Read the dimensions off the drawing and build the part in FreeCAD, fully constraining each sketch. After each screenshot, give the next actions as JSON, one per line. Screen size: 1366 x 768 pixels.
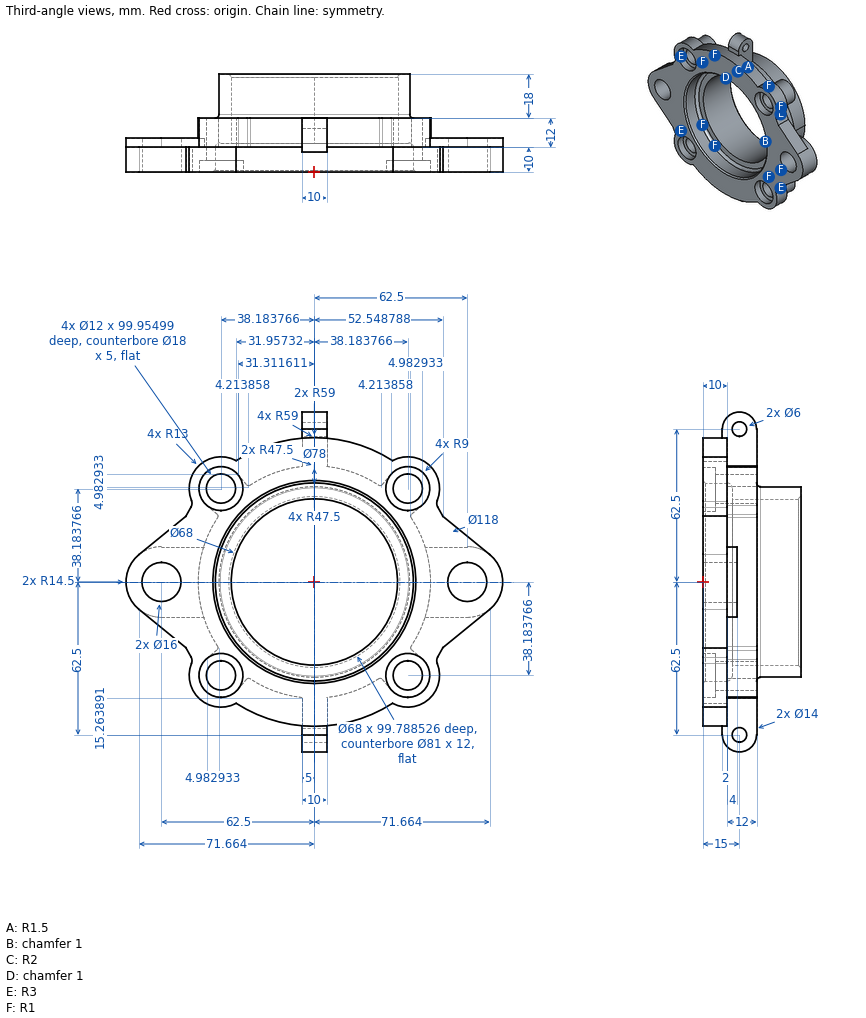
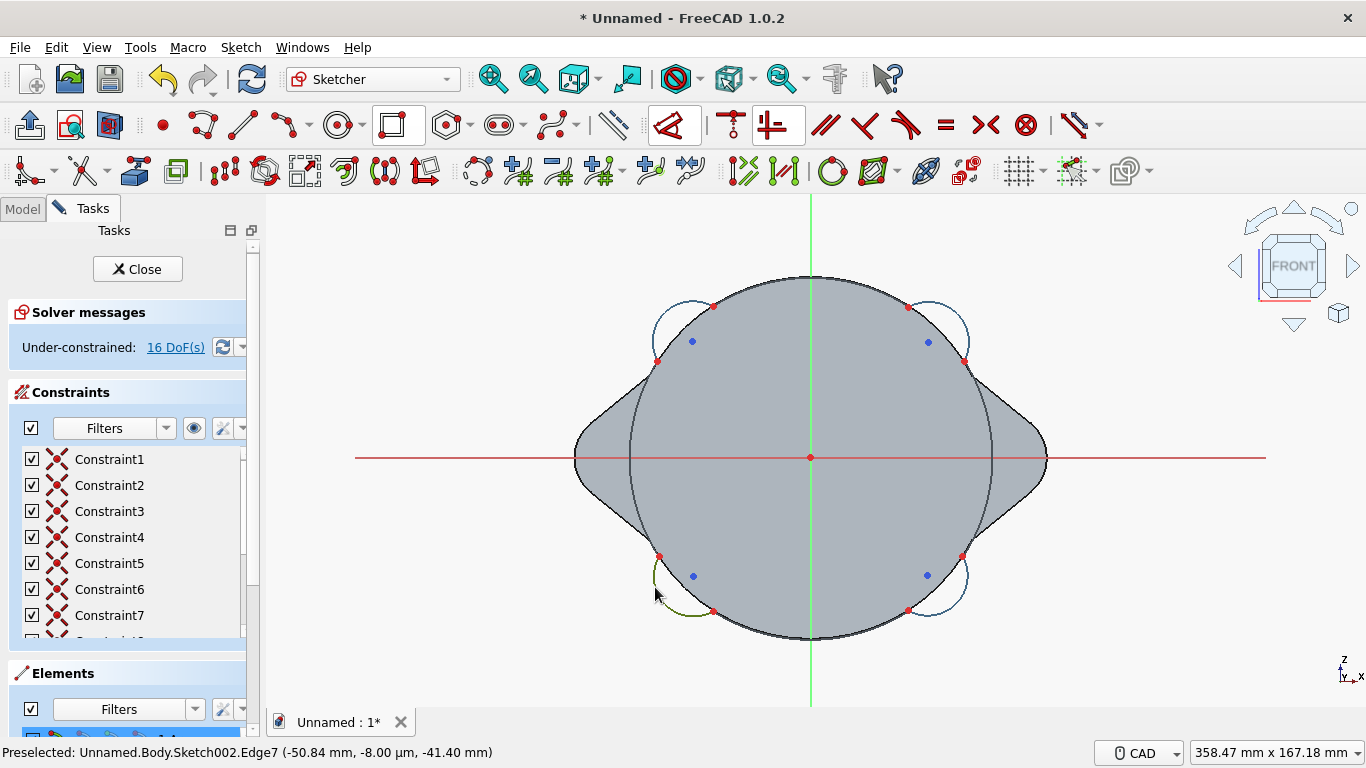
{"action": "left_click", "coordinate": [946, 126]}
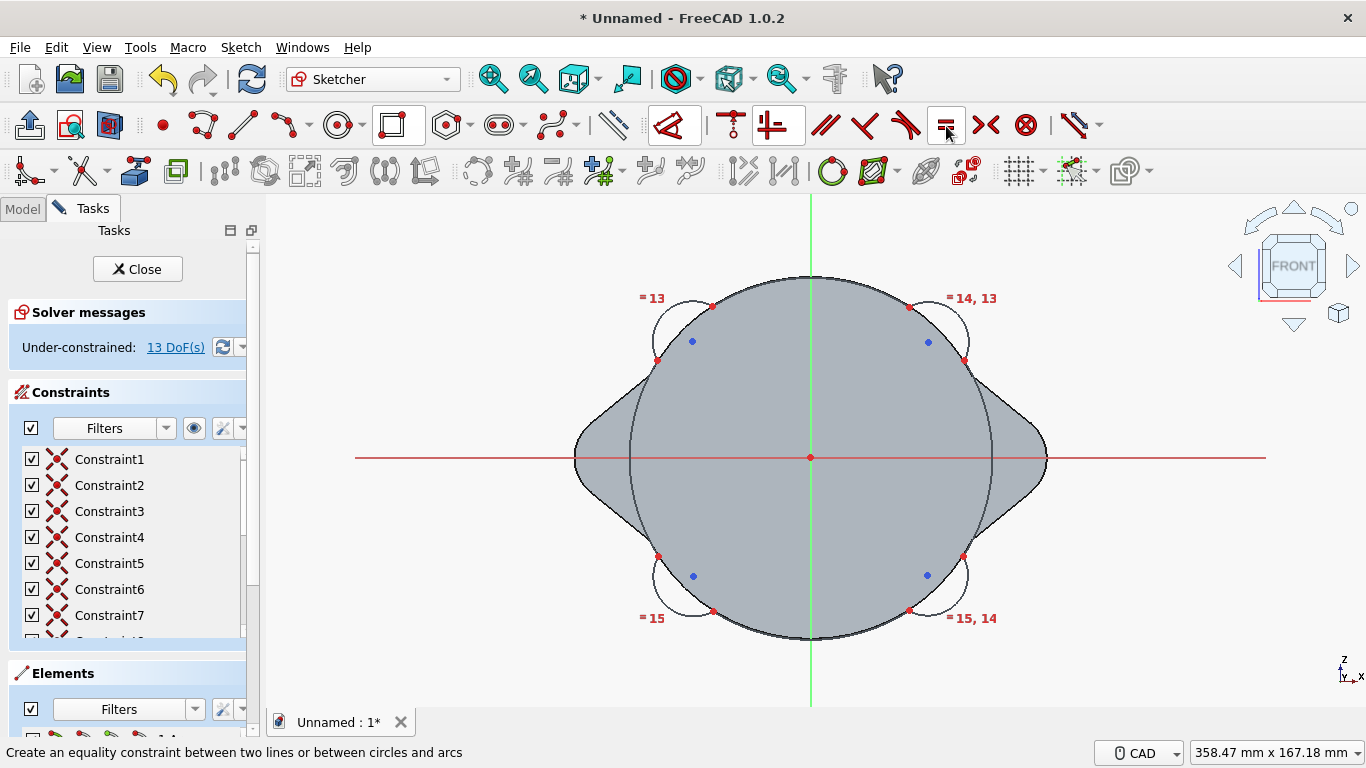
{"action": "left_click", "coordinate": [852, 283]}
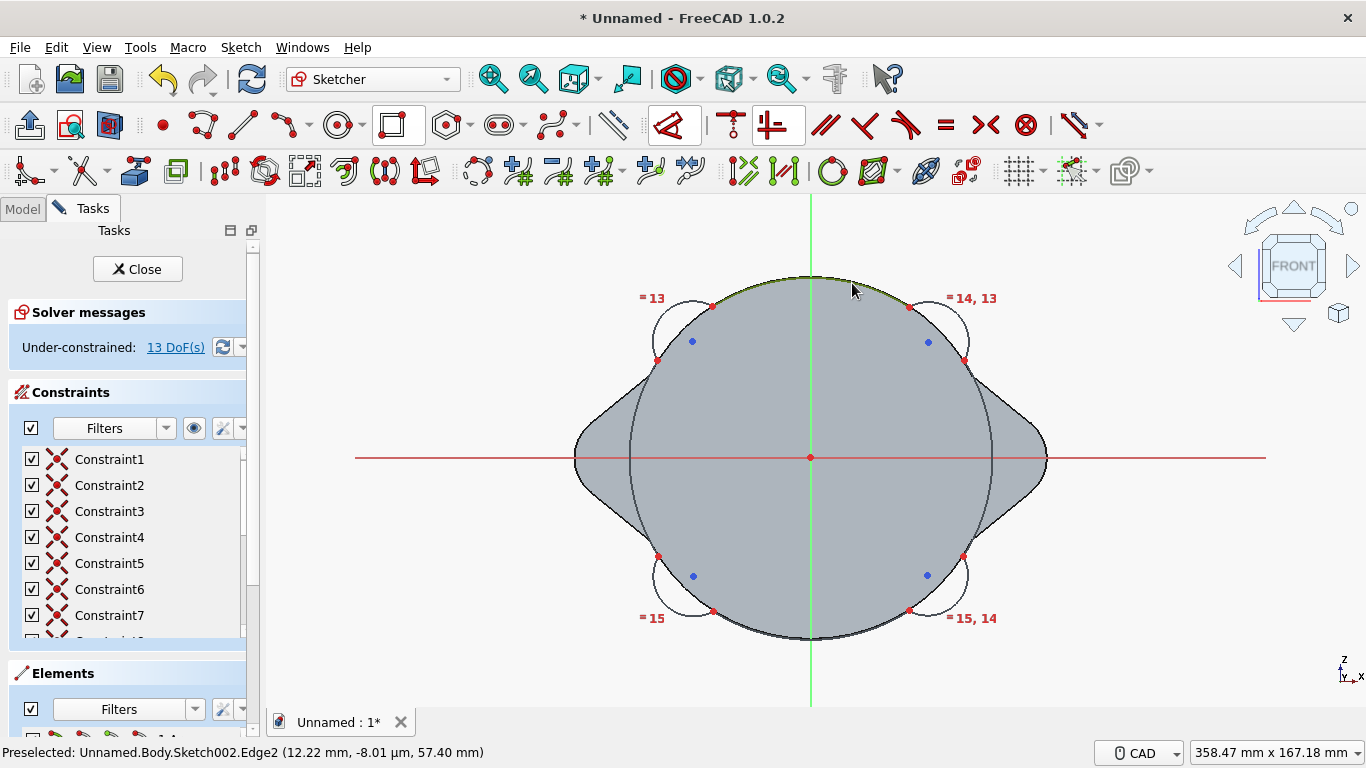
{"action": "left_click", "coordinate": [987, 500]}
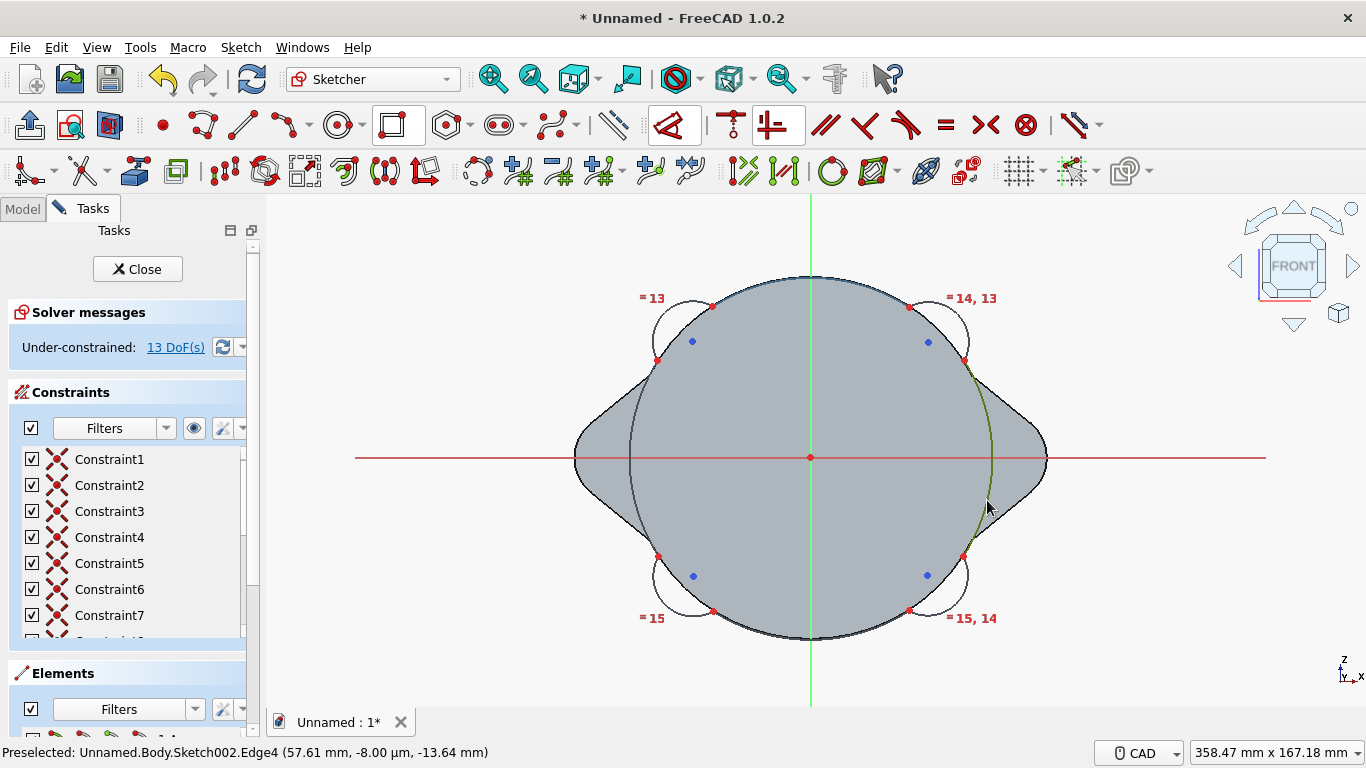
{"action": "left_click", "coordinate": [770, 635]}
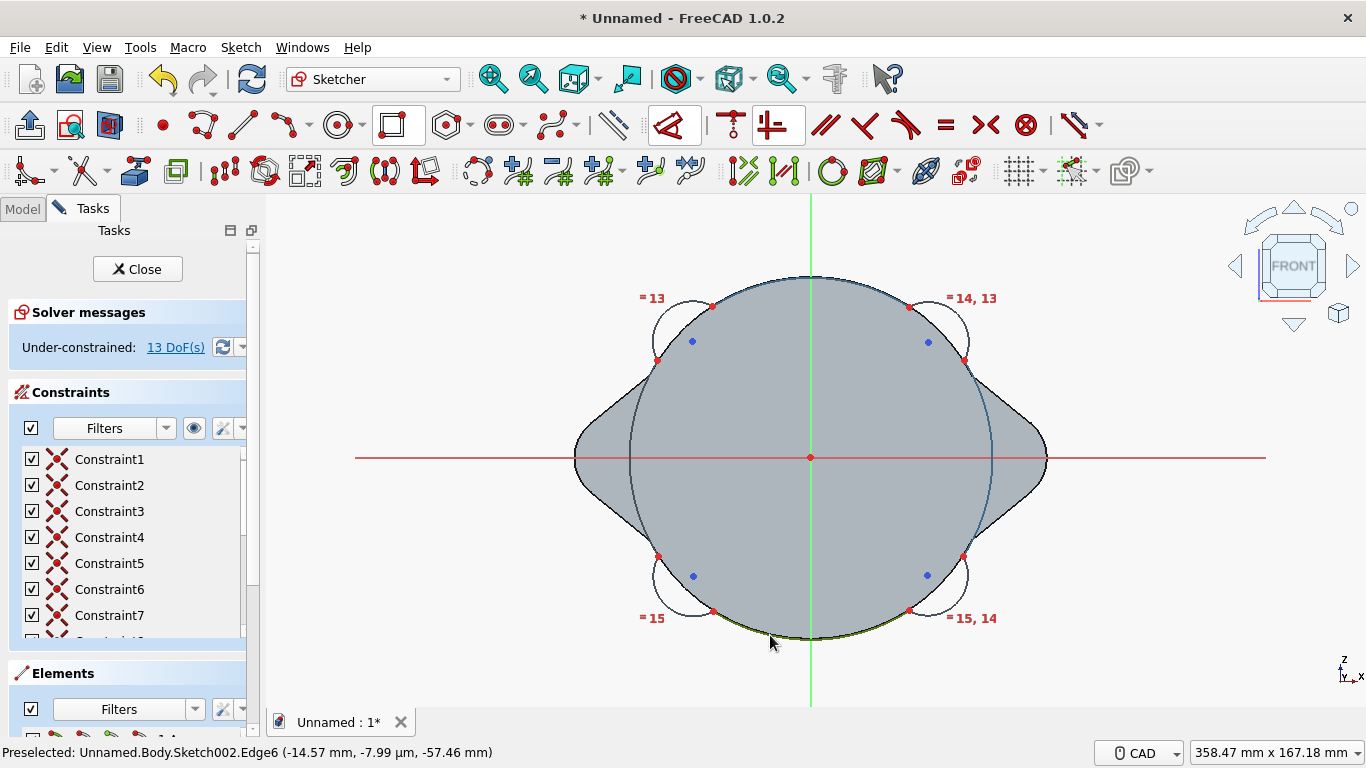
{"action": "left_click", "coordinate": [634, 418]}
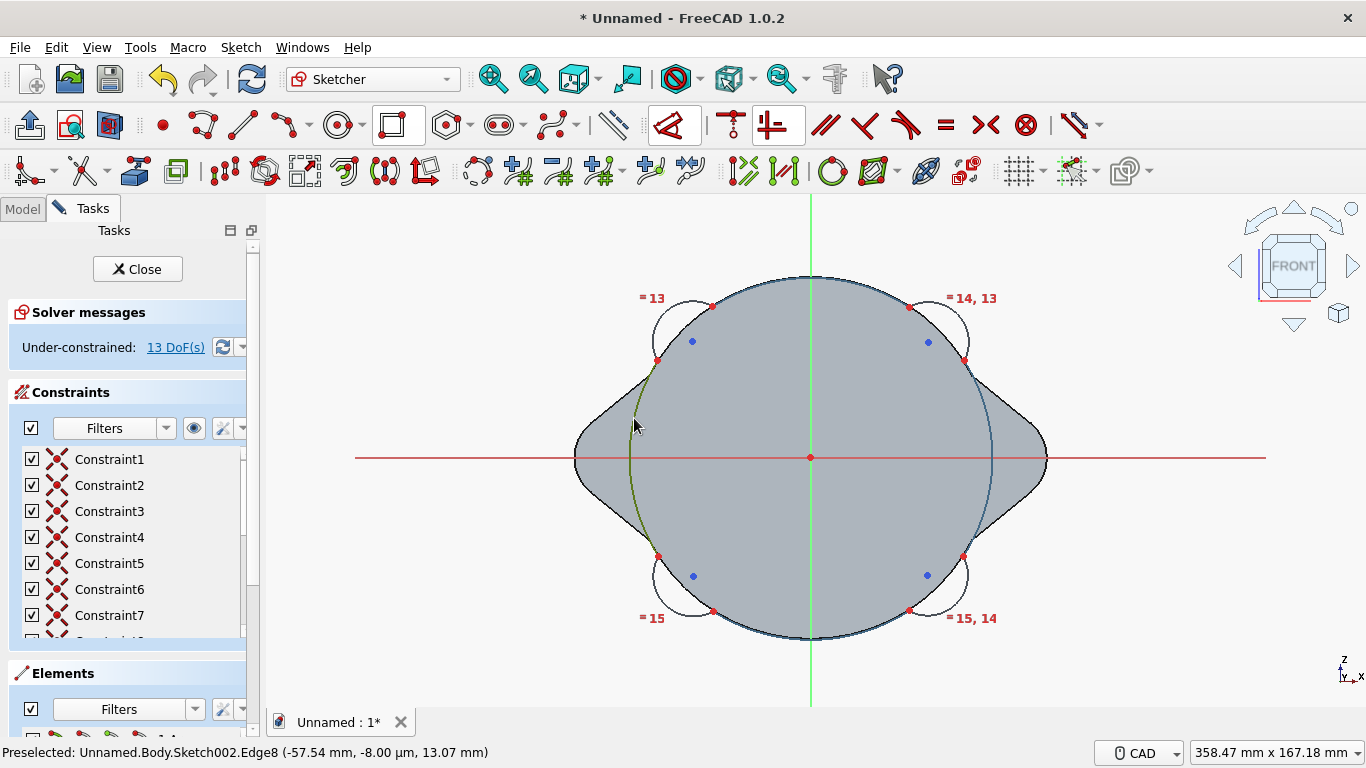
{"action": "left_click", "coordinate": [946, 126]}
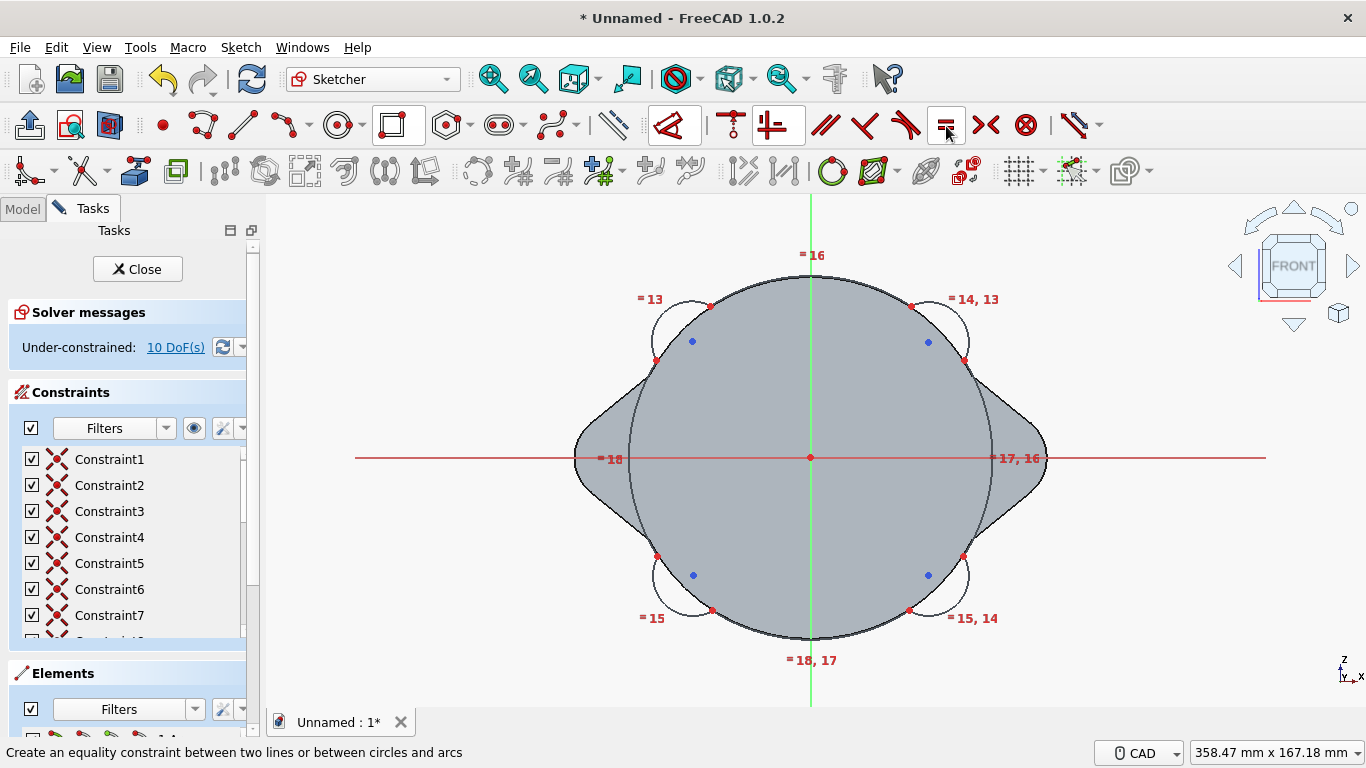
{"action": "left_click", "coordinate": [692, 341]}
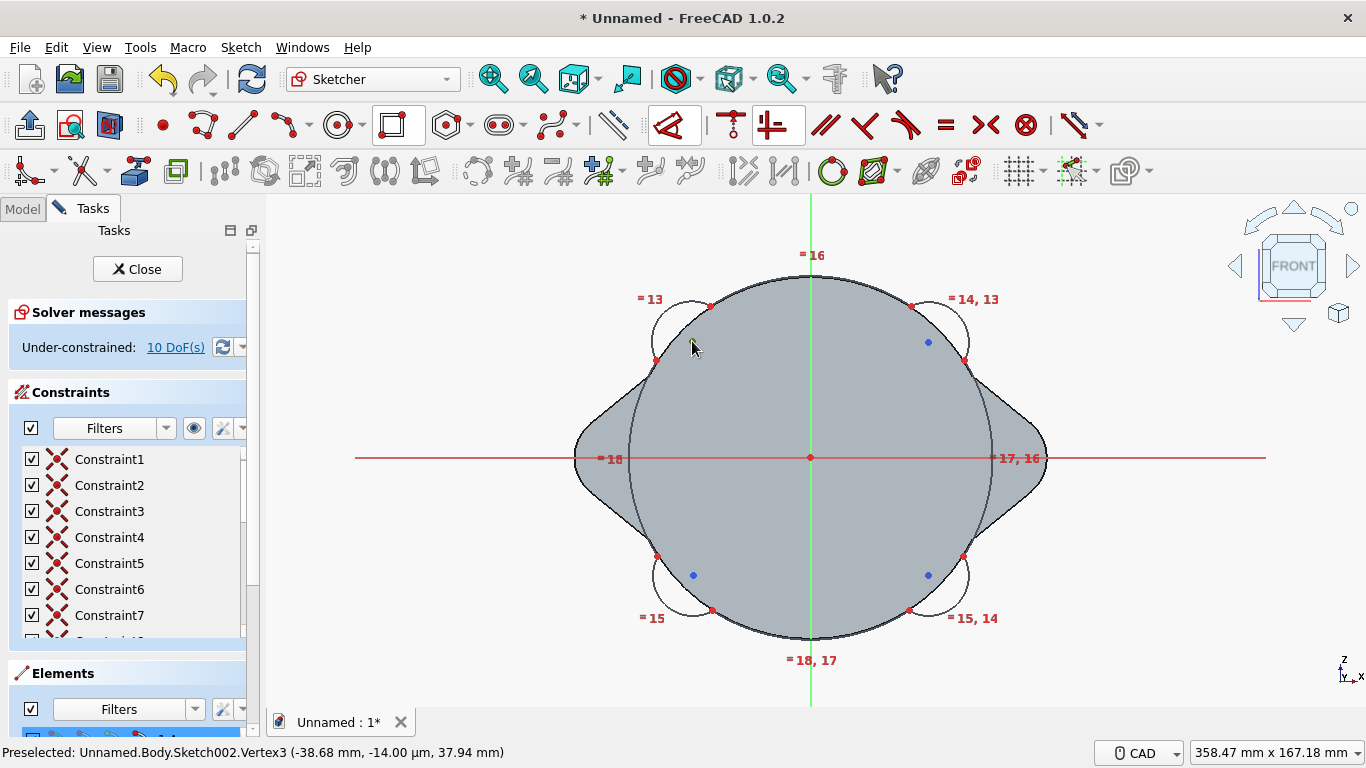
{"action": "left_click", "coordinate": [929, 342]}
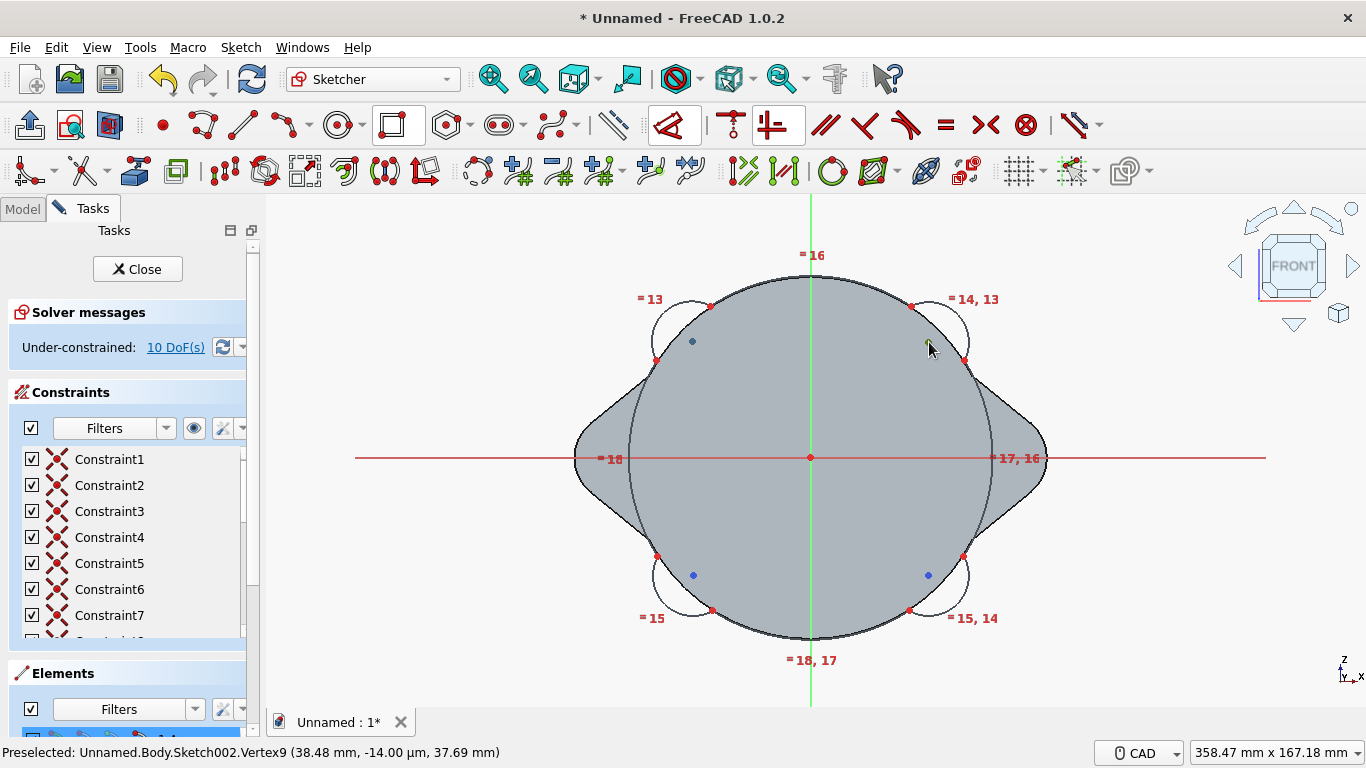
{"action": "left_click", "coordinate": [811, 581]}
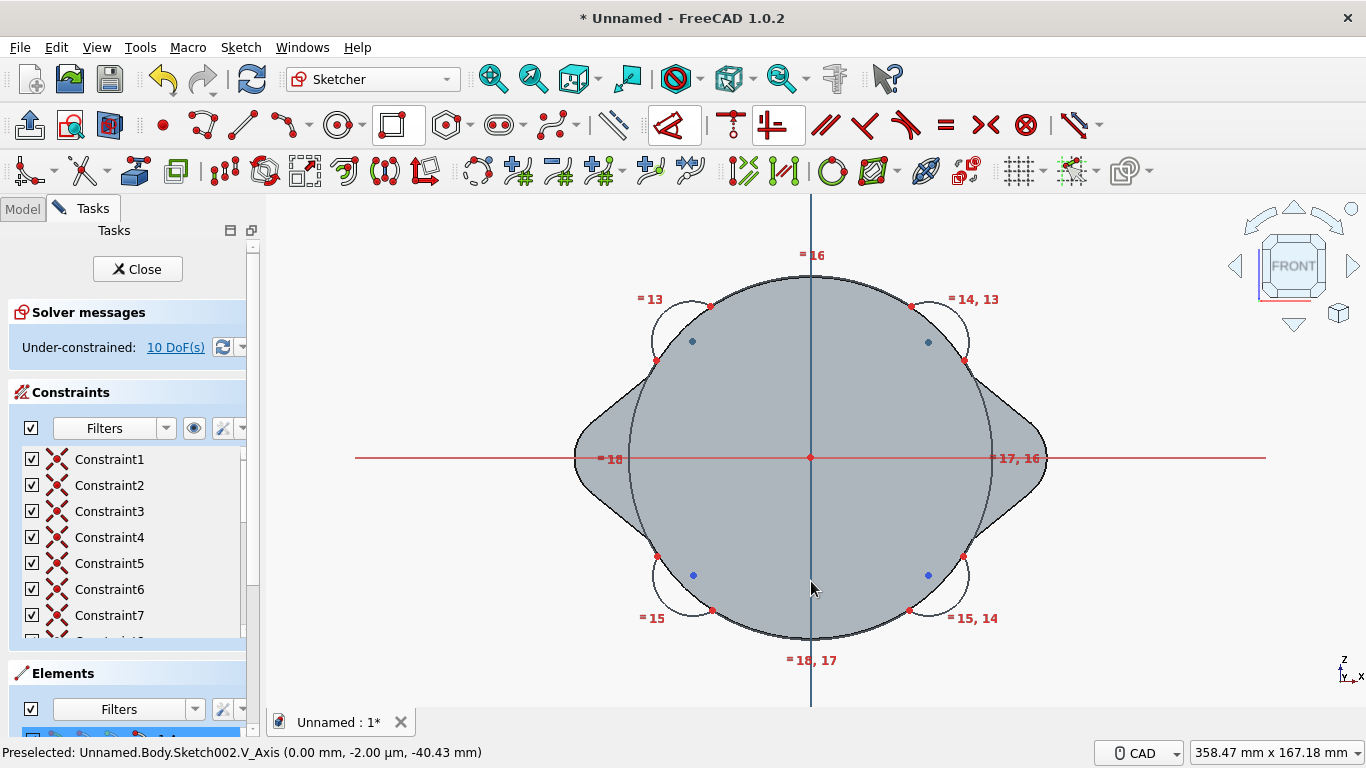
{"action": "left_click", "coordinate": [986, 126]}